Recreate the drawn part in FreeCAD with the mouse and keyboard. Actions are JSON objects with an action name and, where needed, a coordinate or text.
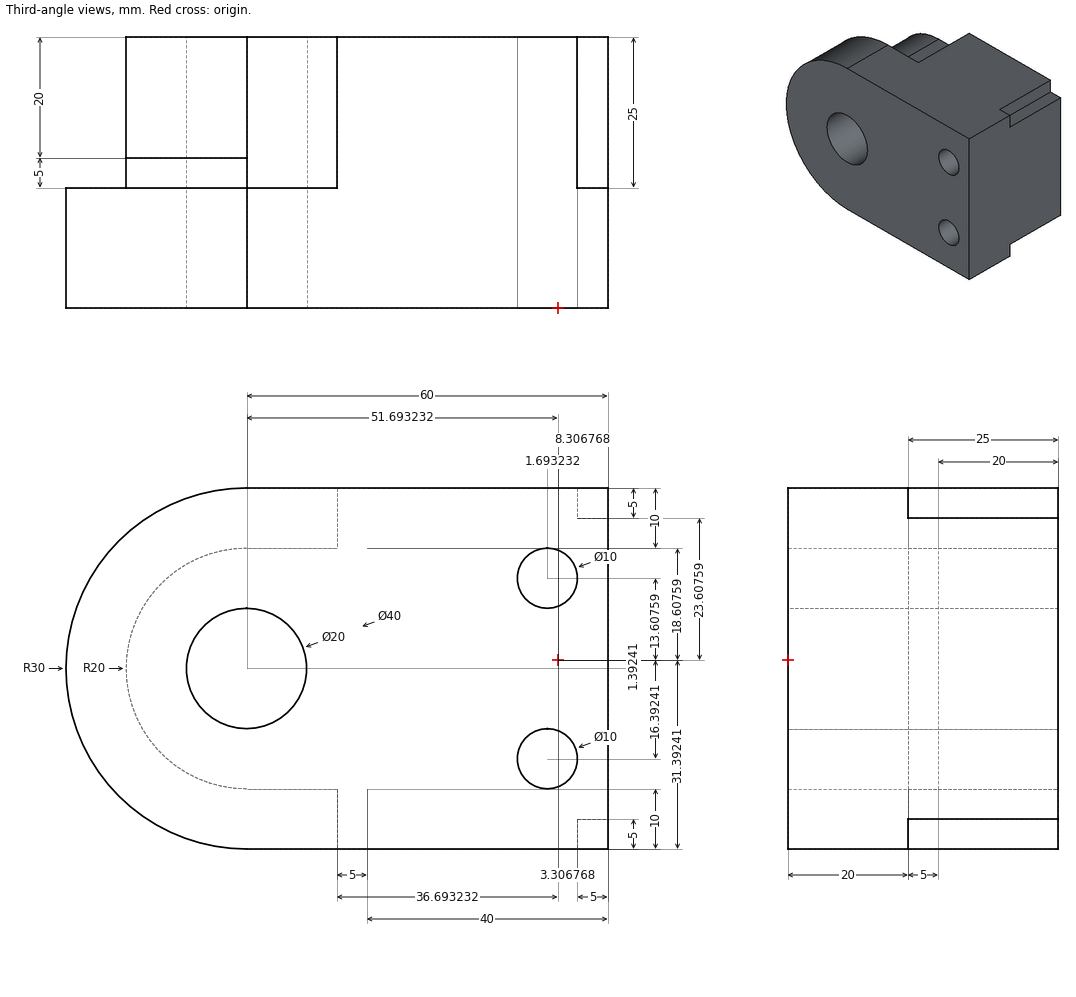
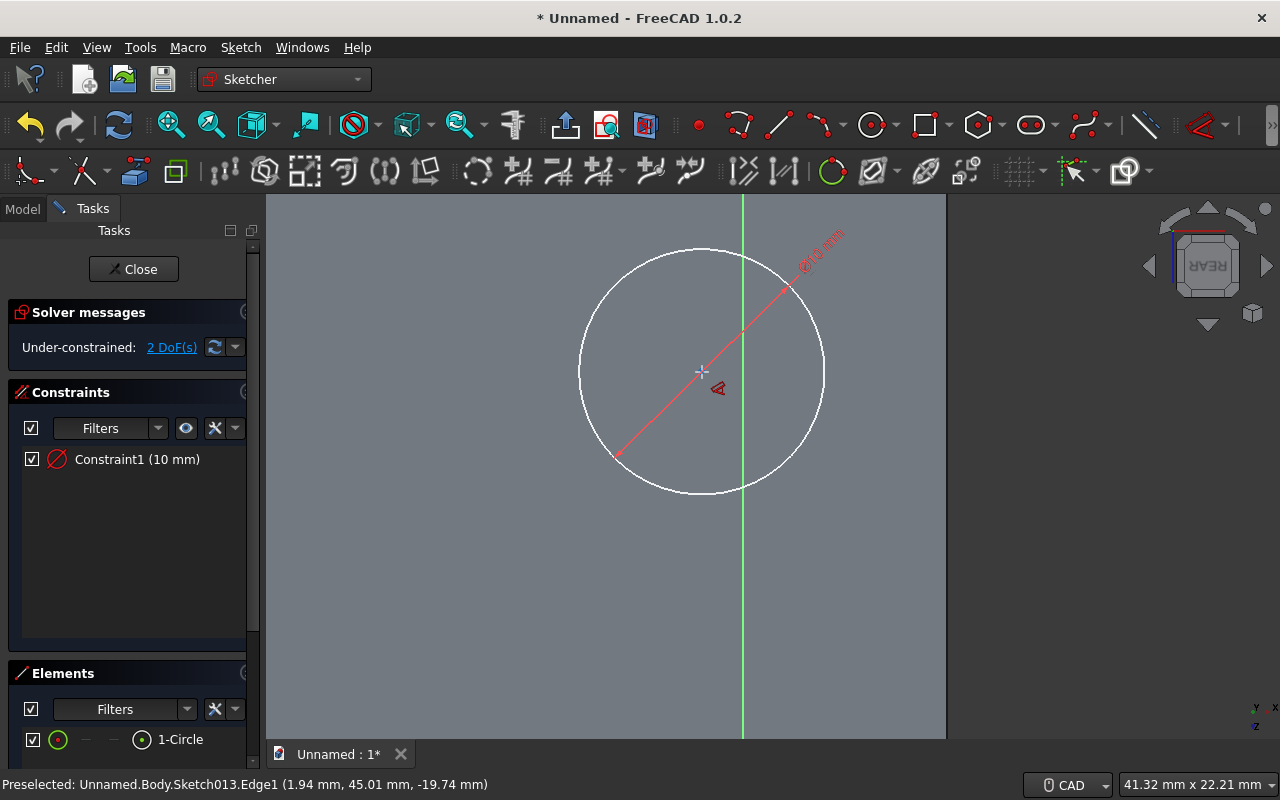
{"action": "left_click", "coordinate": [702, 372]}
{"action": "left_click", "coordinate": [723, 338]}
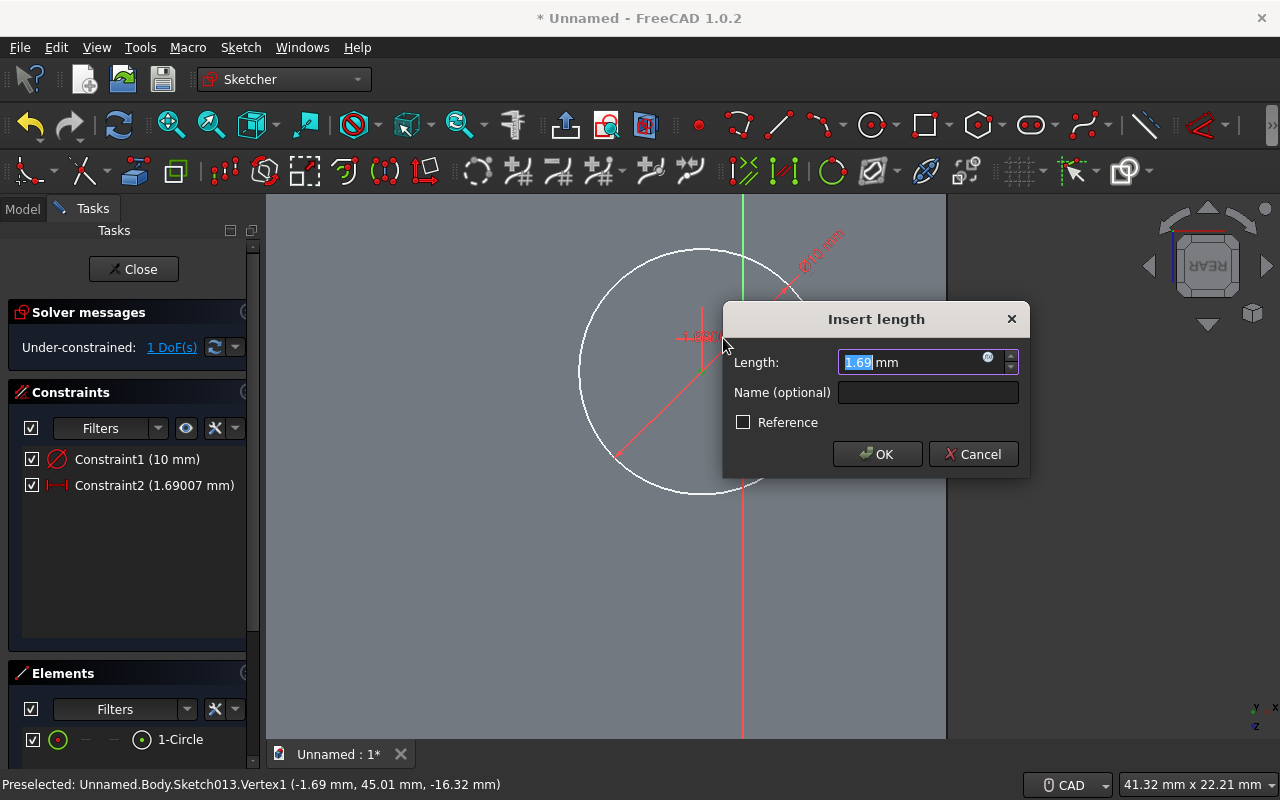
{"action": "type", "text": "1.693232"}
{"action": "key", "text": "Return"}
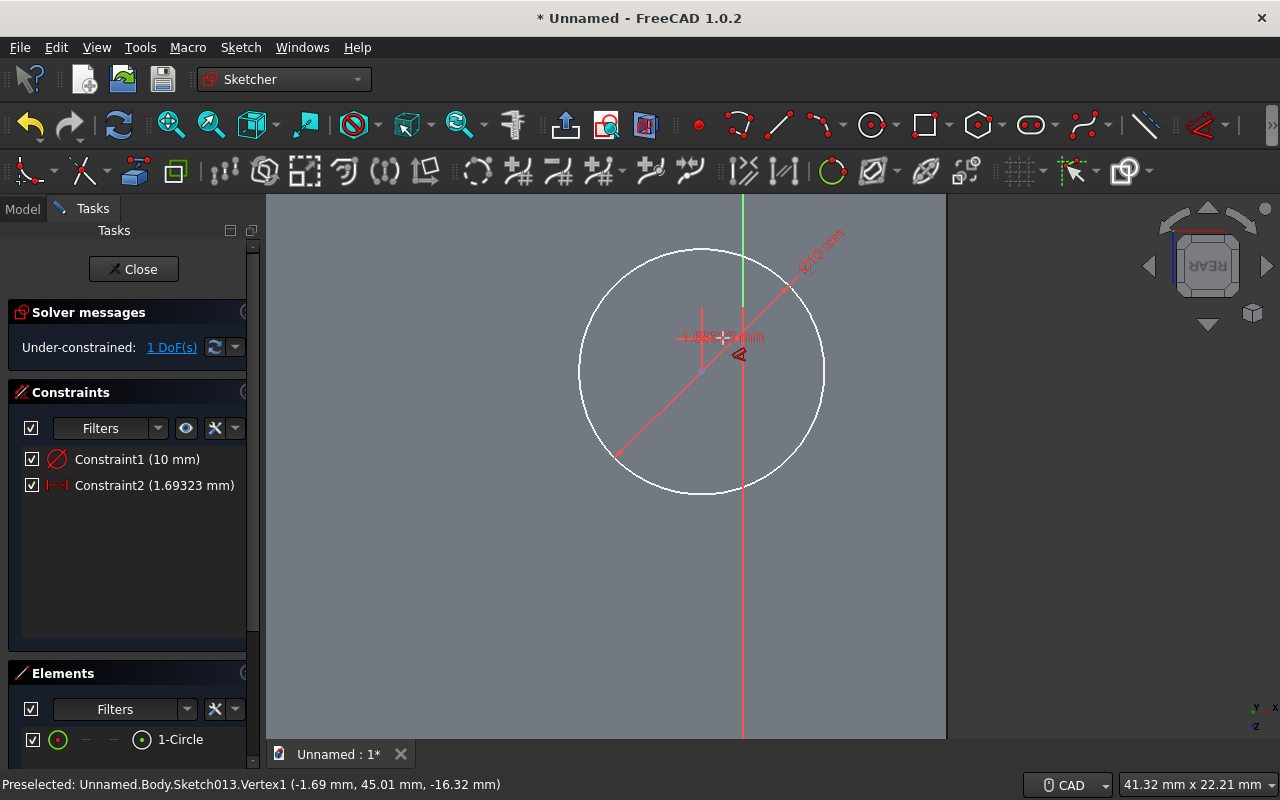
{"action": "left_click", "coordinate": [702, 372]}
{"action": "left_click", "coordinate": [777, 541]}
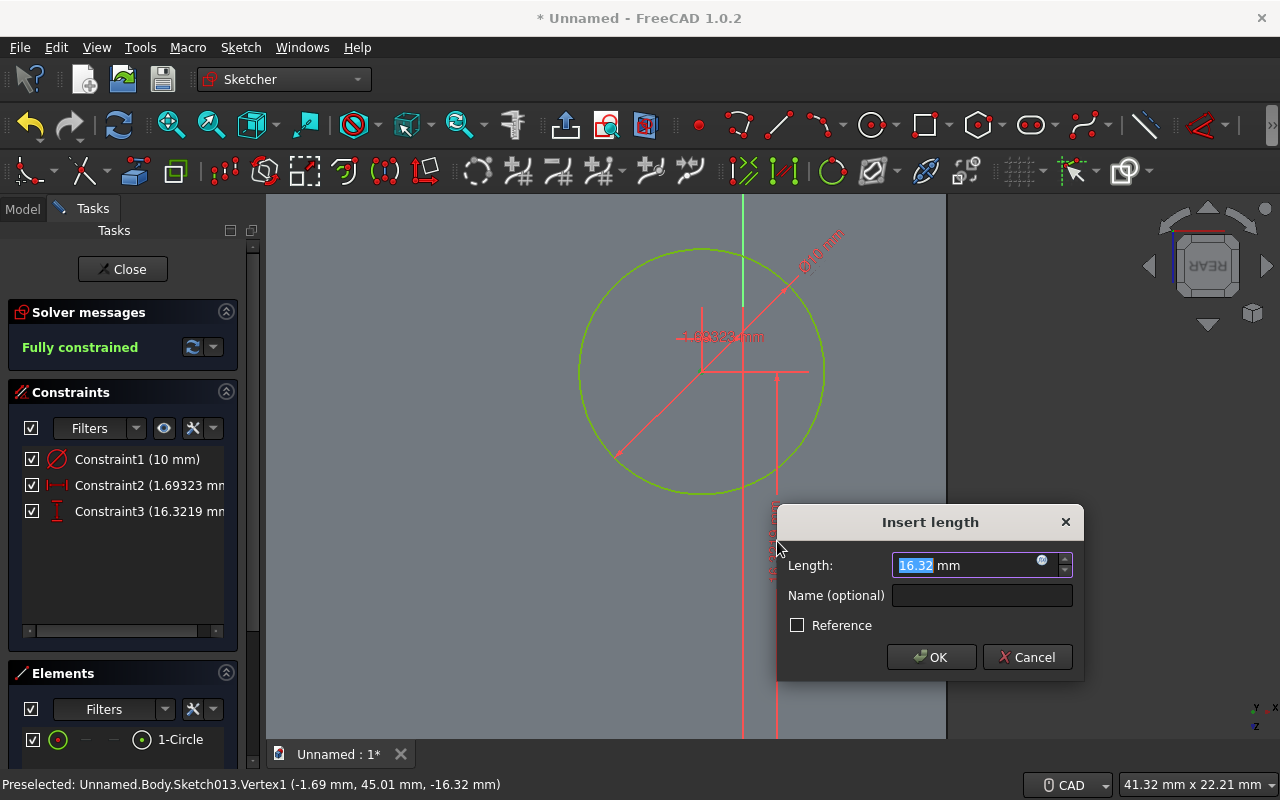
{"action": "type", "text": "16.39241"}
{"action": "key", "text": "Return"}
{"action": "key", "text": "Escape"}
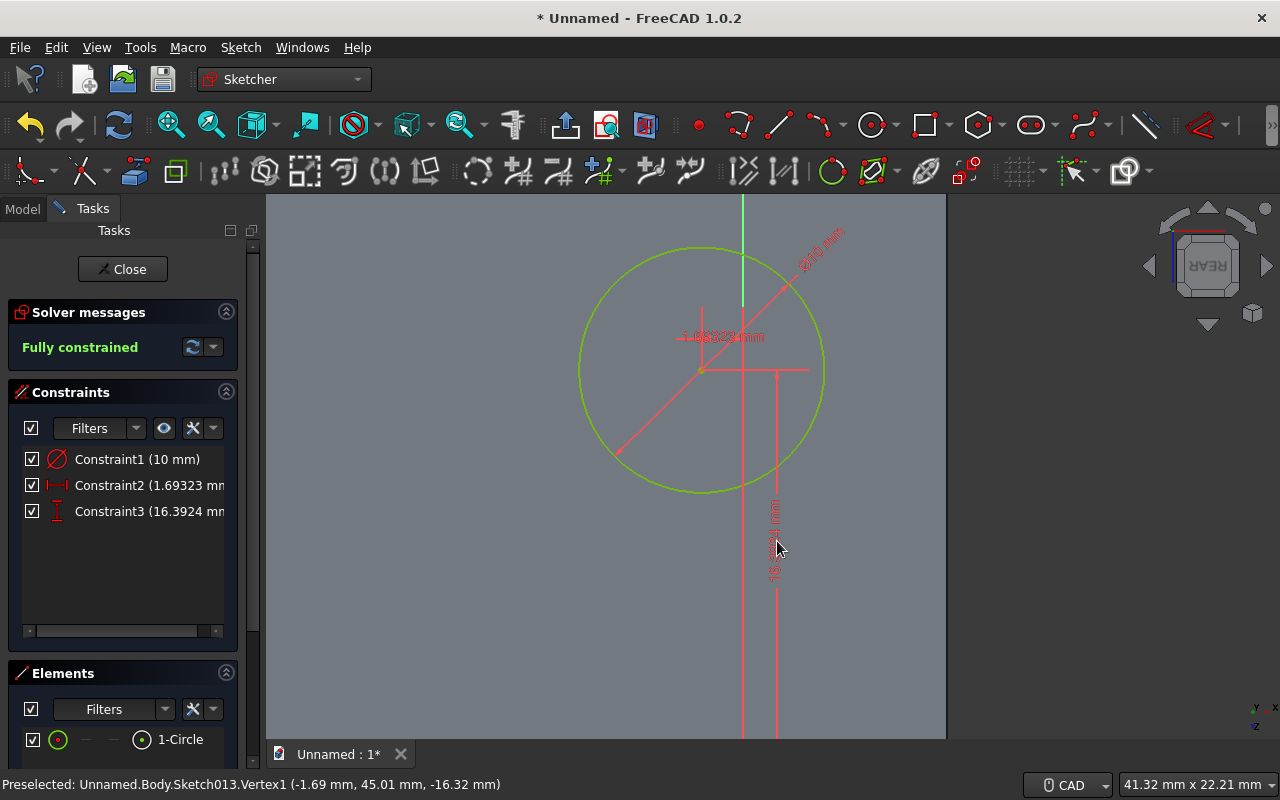
{"action": "left_click", "coordinate": [123, 269]}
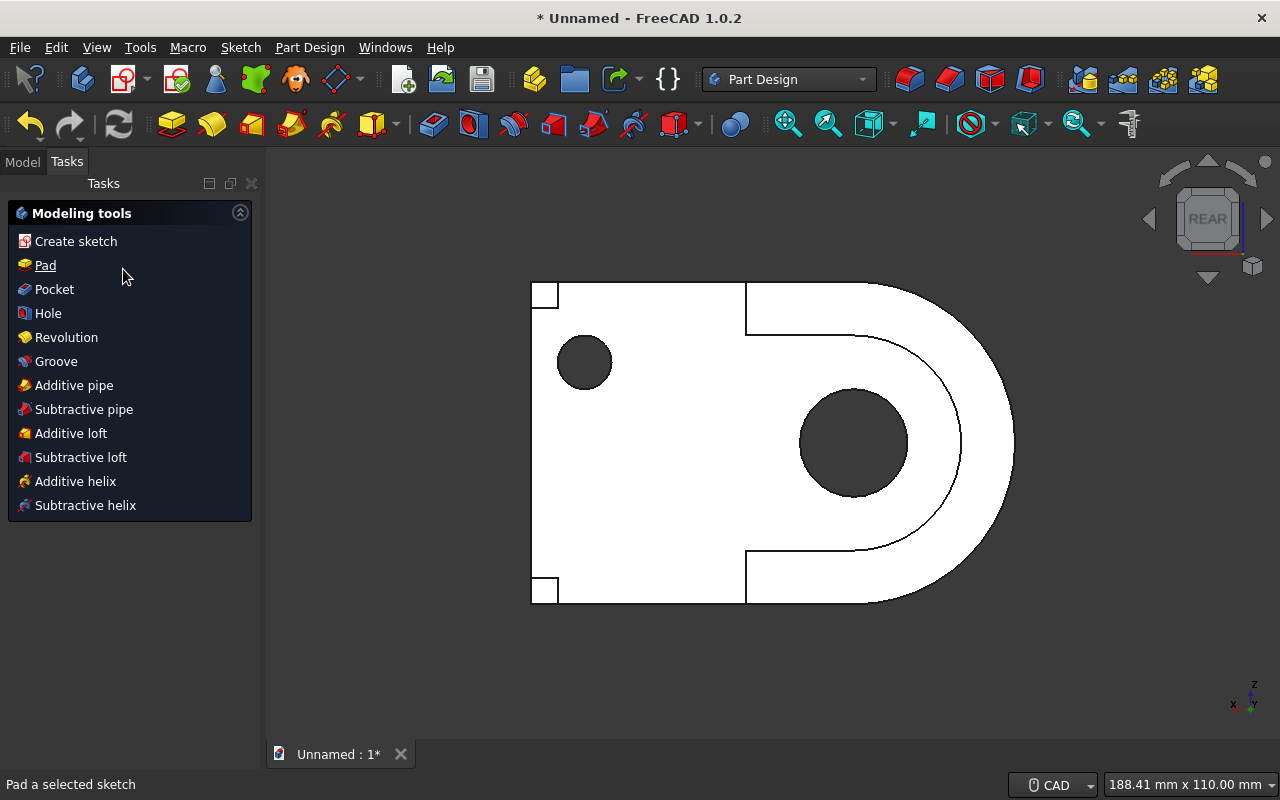
{"action": "left_click", "coordinate": [434, 124]}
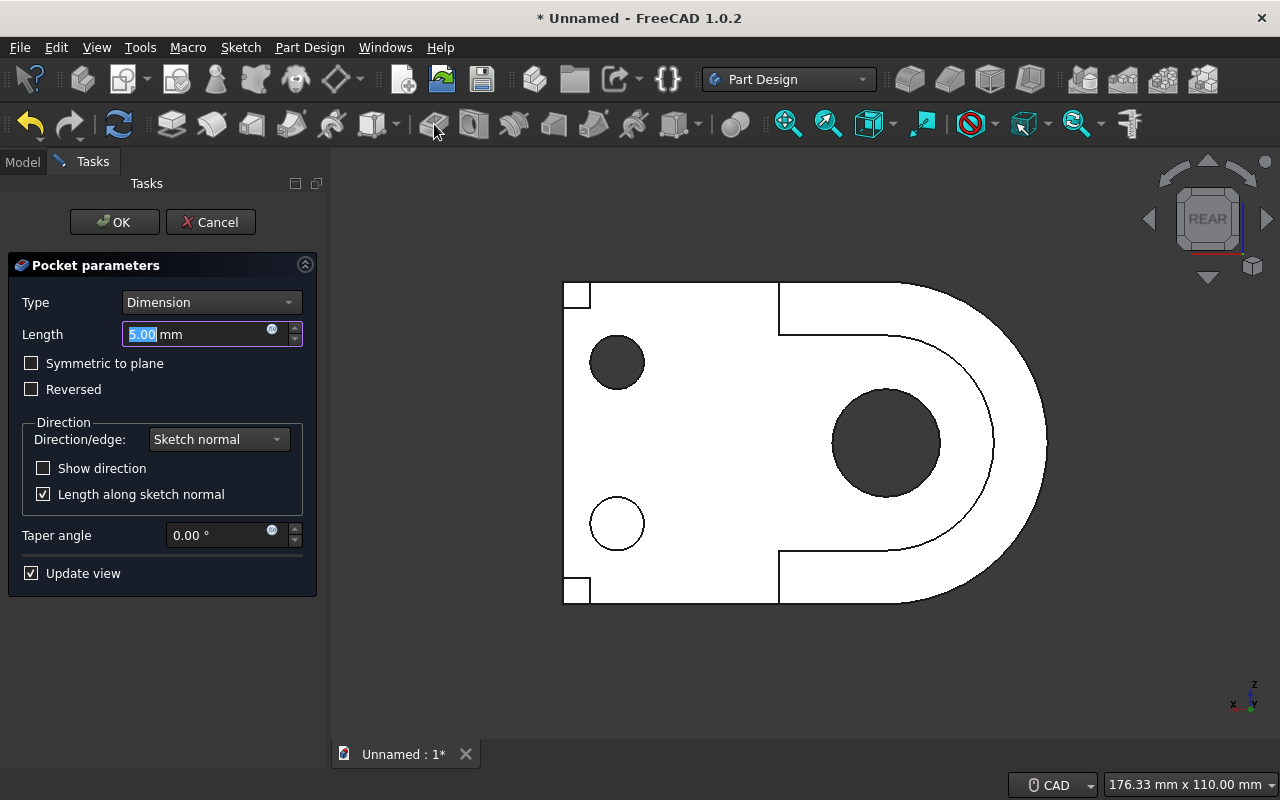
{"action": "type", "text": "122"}
{"action": "key", "text": "Tab"}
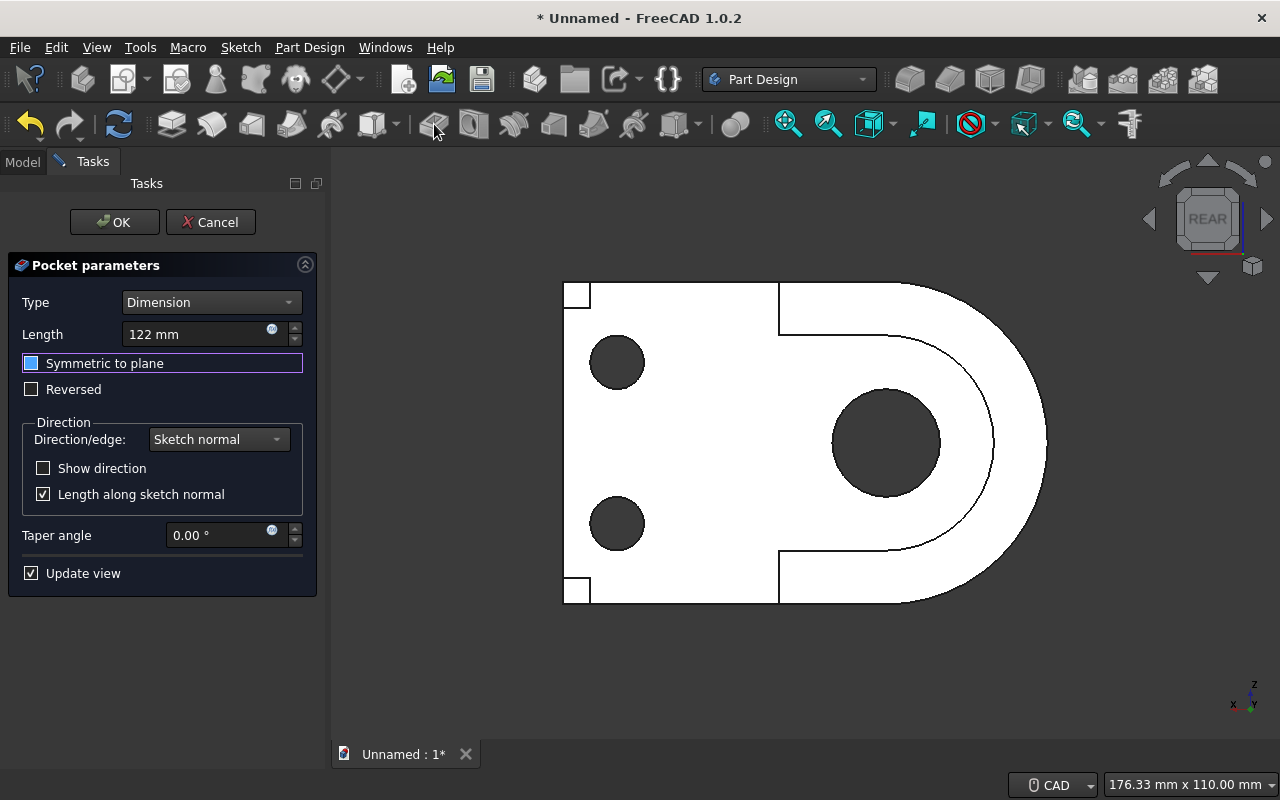
{"action": "left_click", "coordinate": [115, 222]}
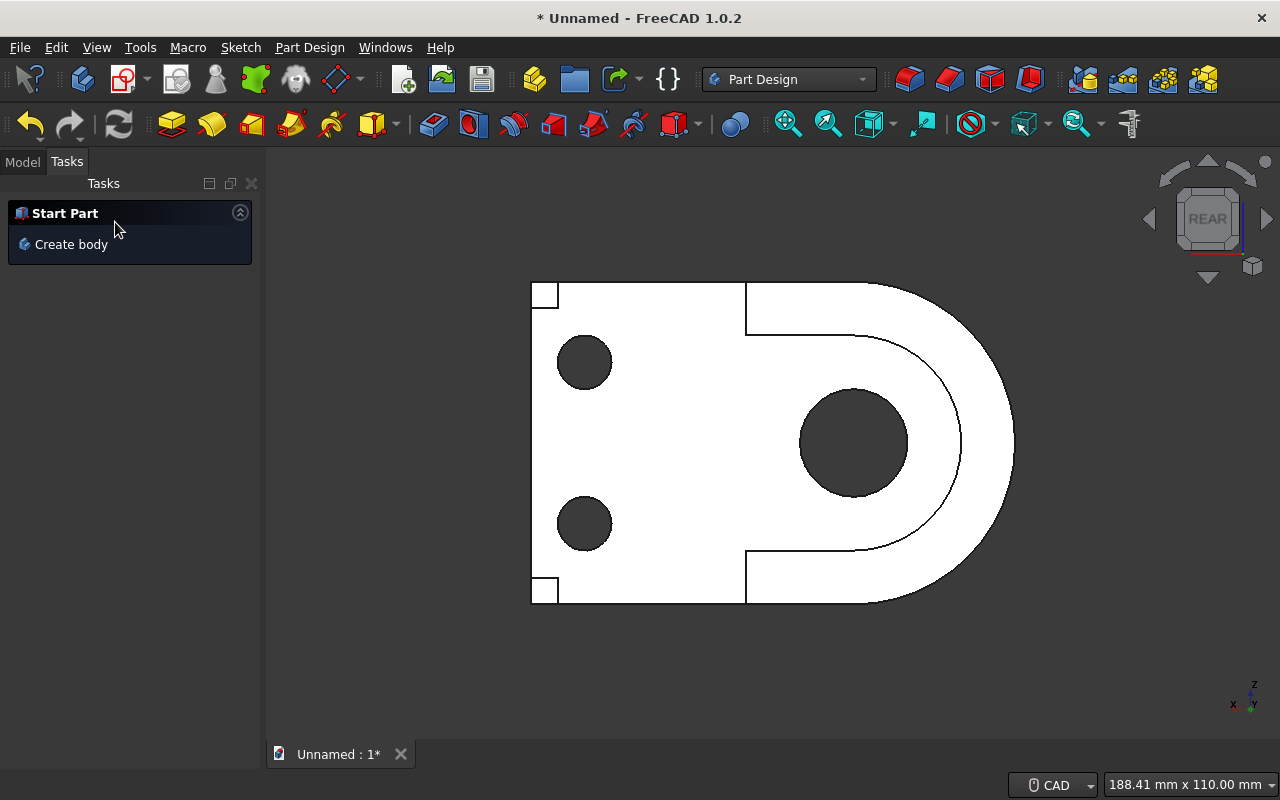
{"action": "left_click", "coordinate": [804, 304]}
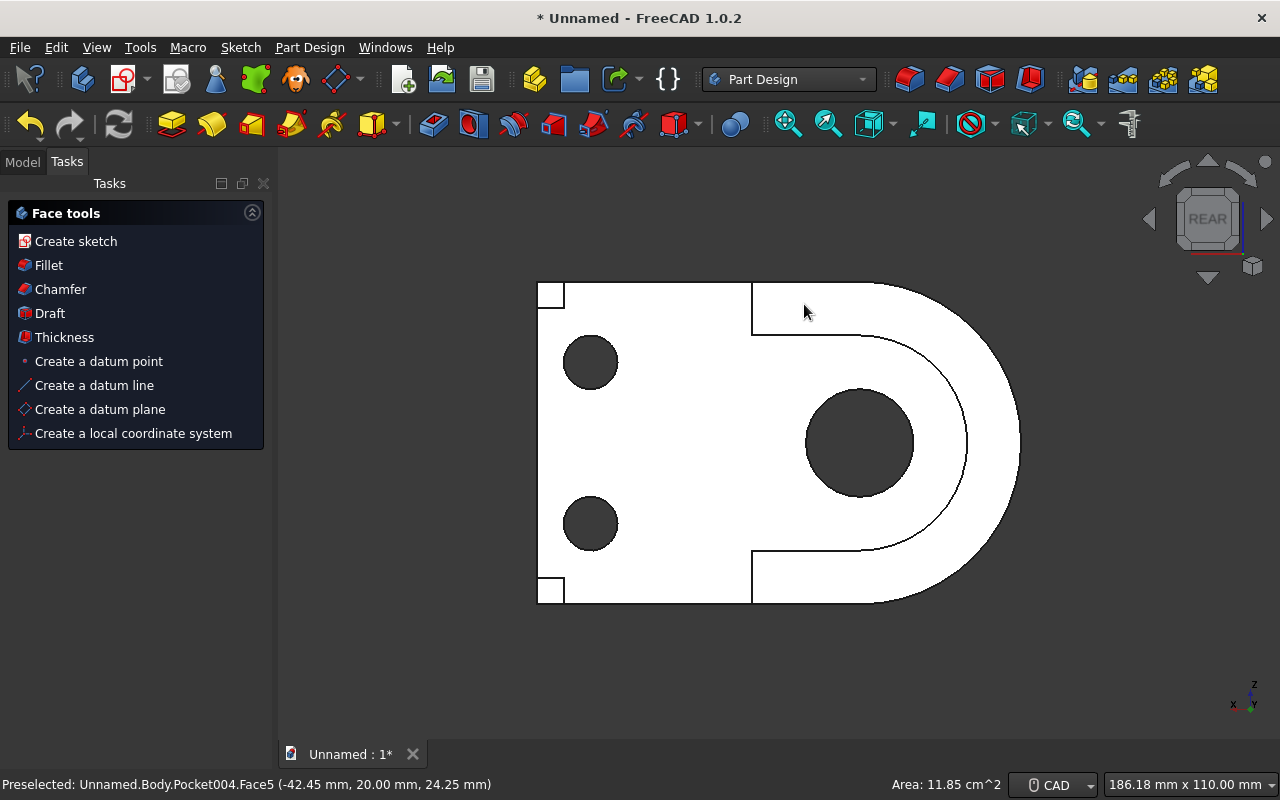
{"action": "left_click", "coordinate": [124, 80]}